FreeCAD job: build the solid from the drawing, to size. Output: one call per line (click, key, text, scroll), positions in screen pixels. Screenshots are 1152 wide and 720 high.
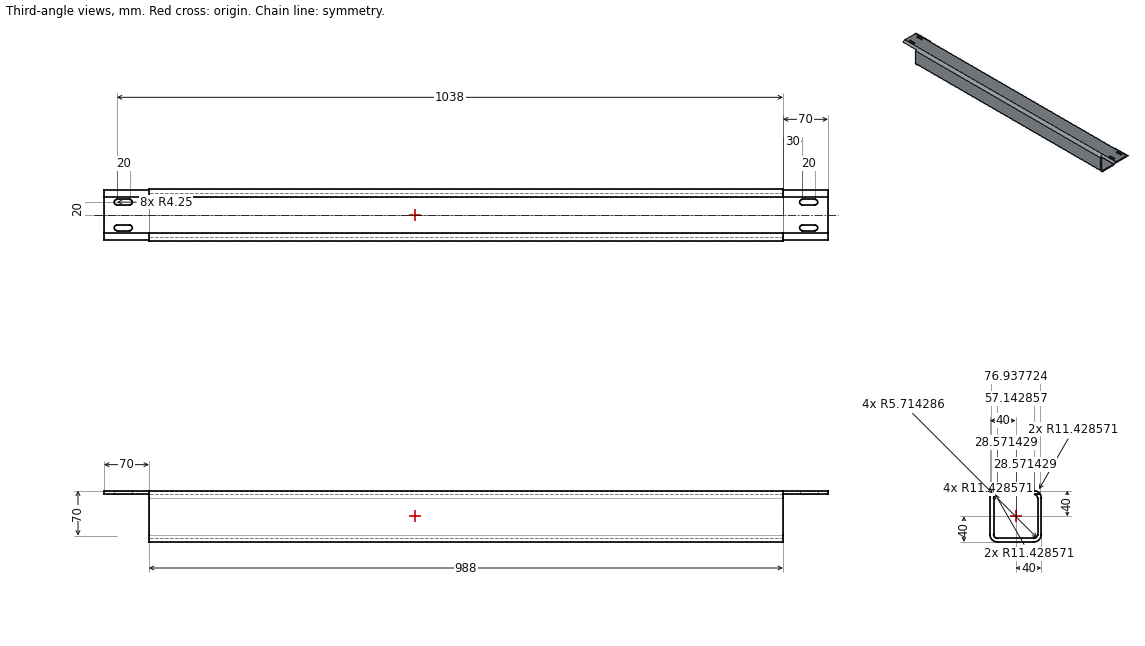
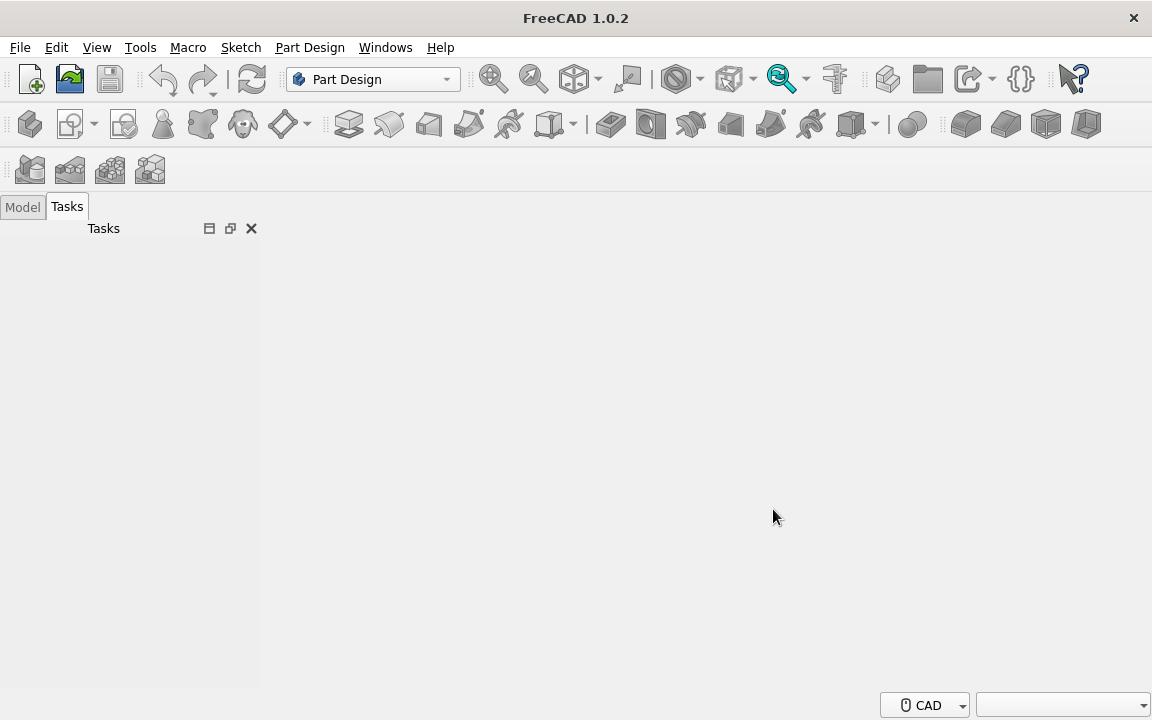
key(ctrl+n)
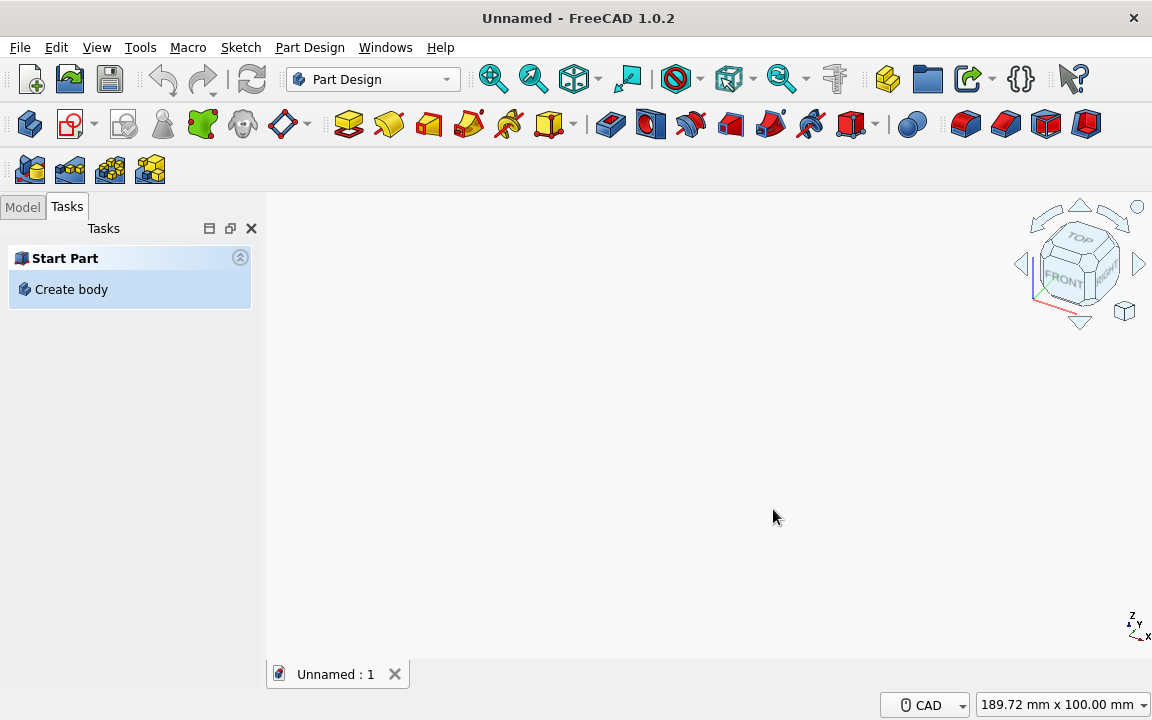
click(30, 124)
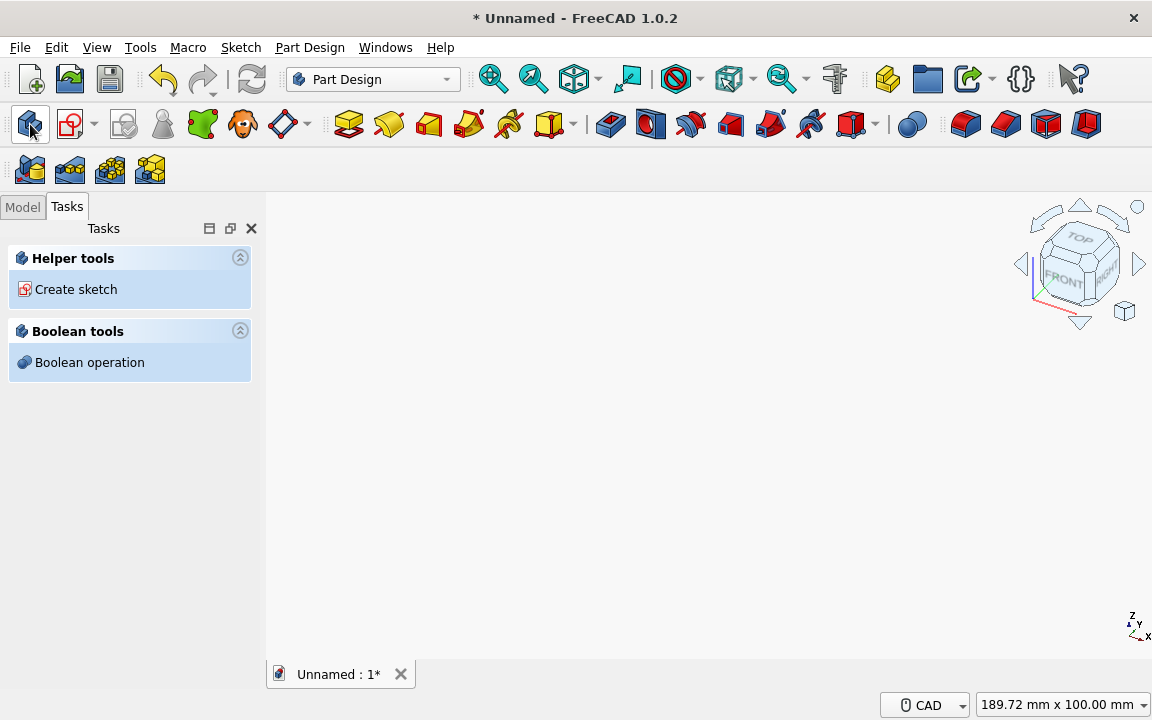
click(23, 206)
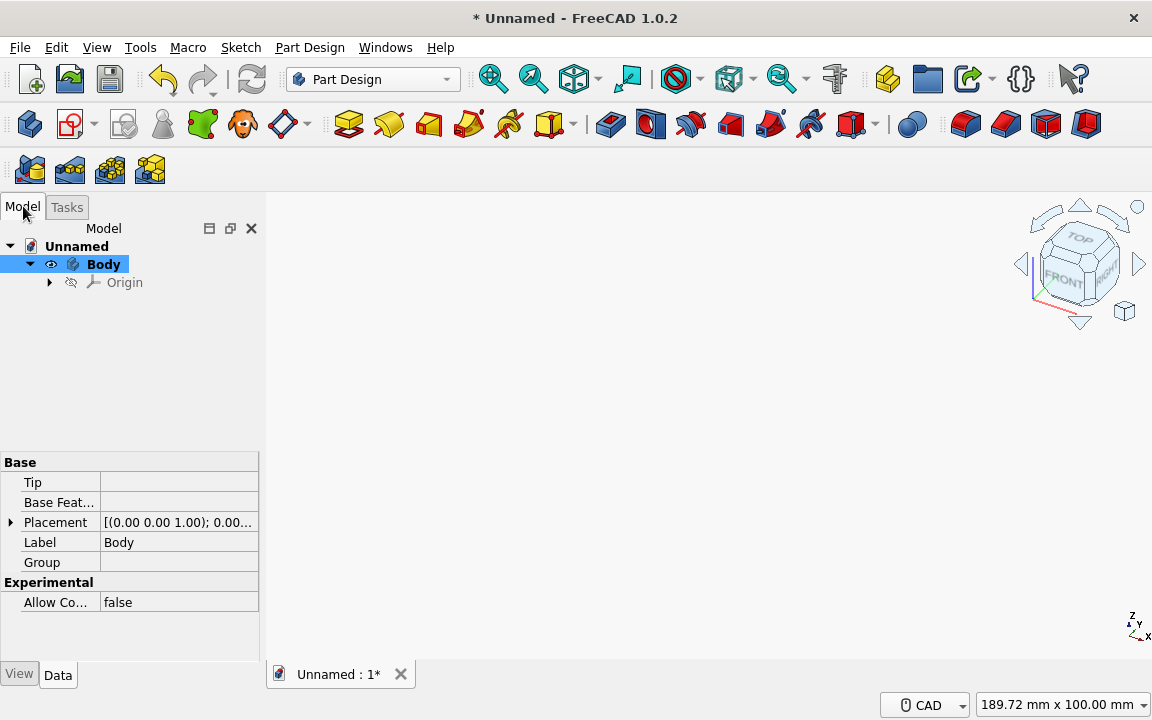
click(50, 282)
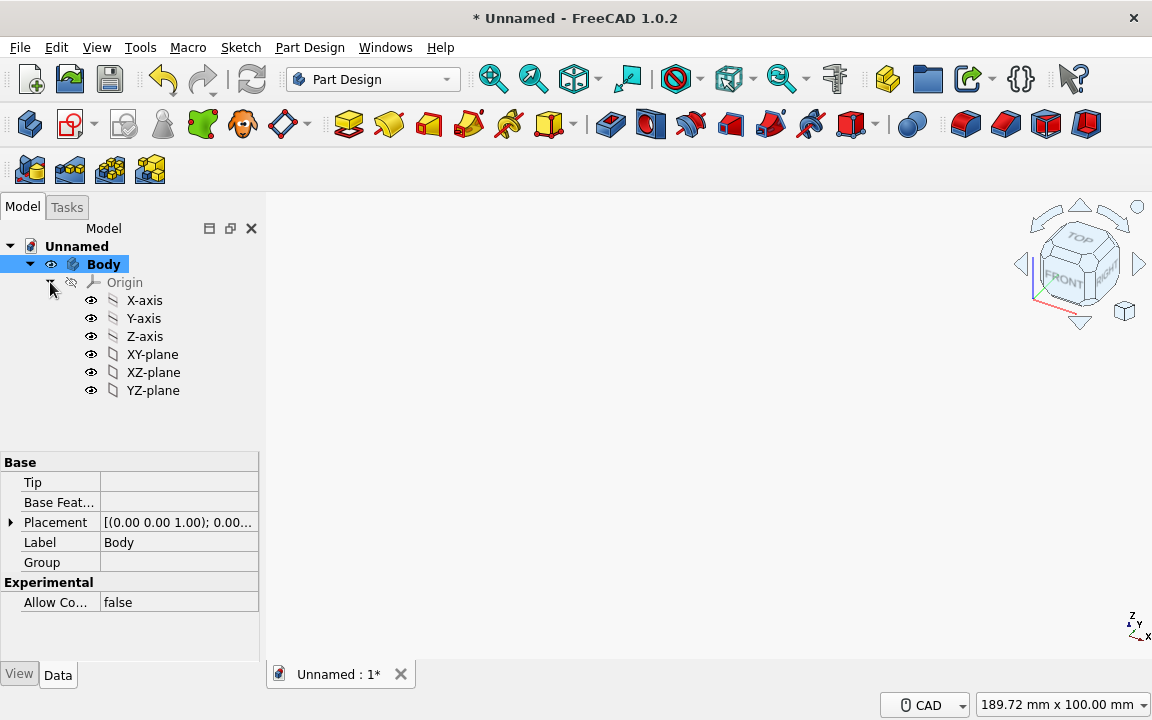
click(136, 390)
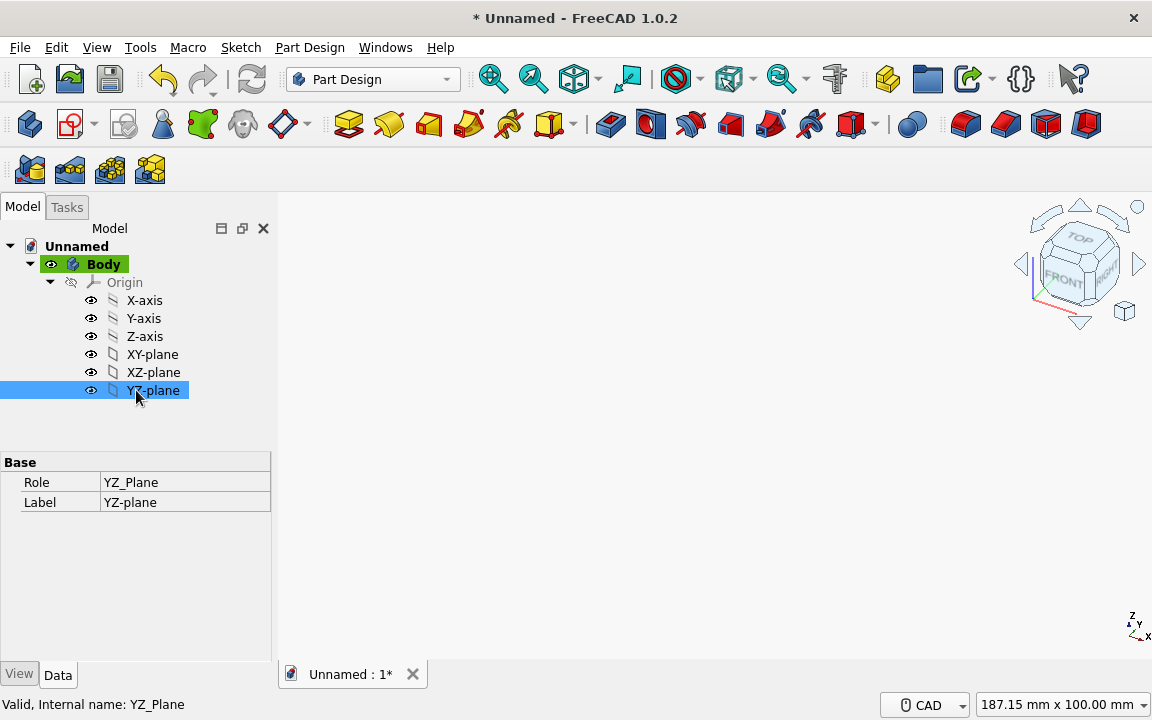
click(284, 124)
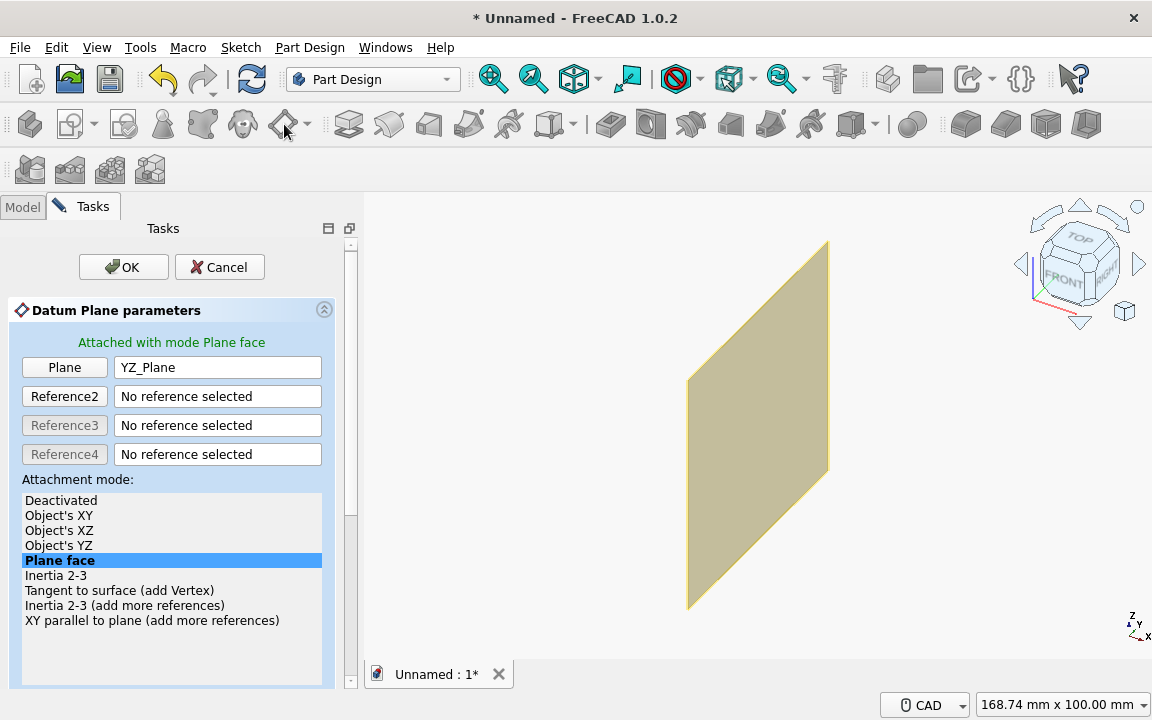
scroll(351, 463, down, 3)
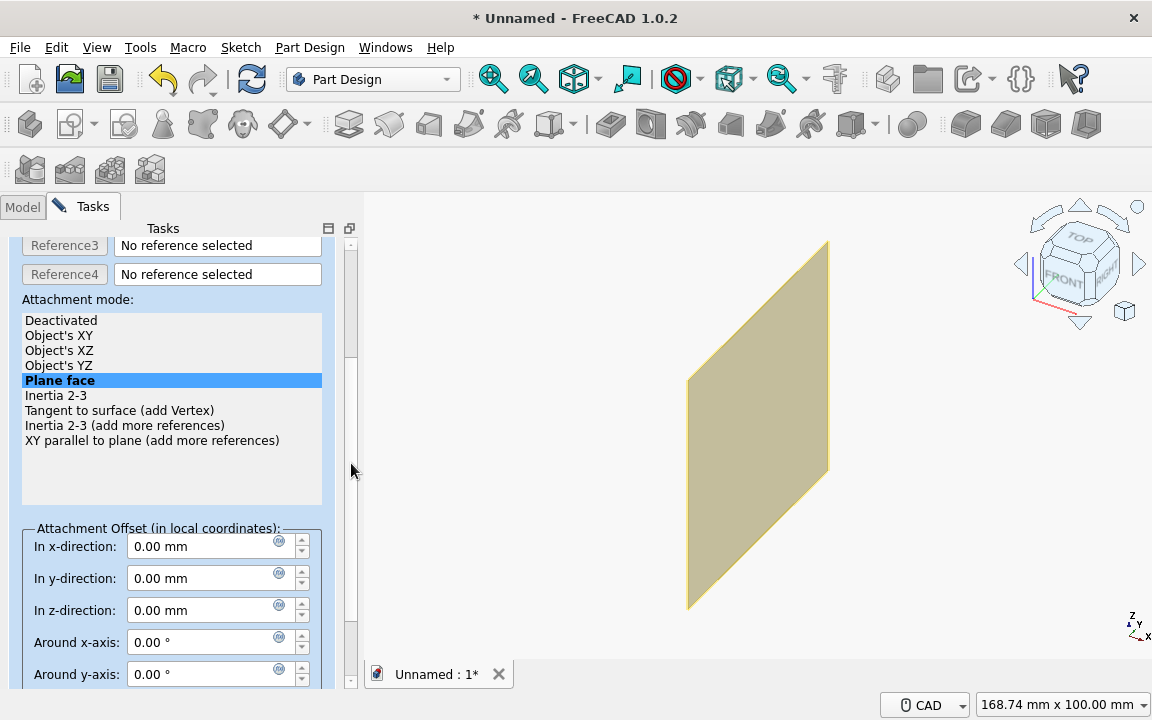
triple_click(210, 610)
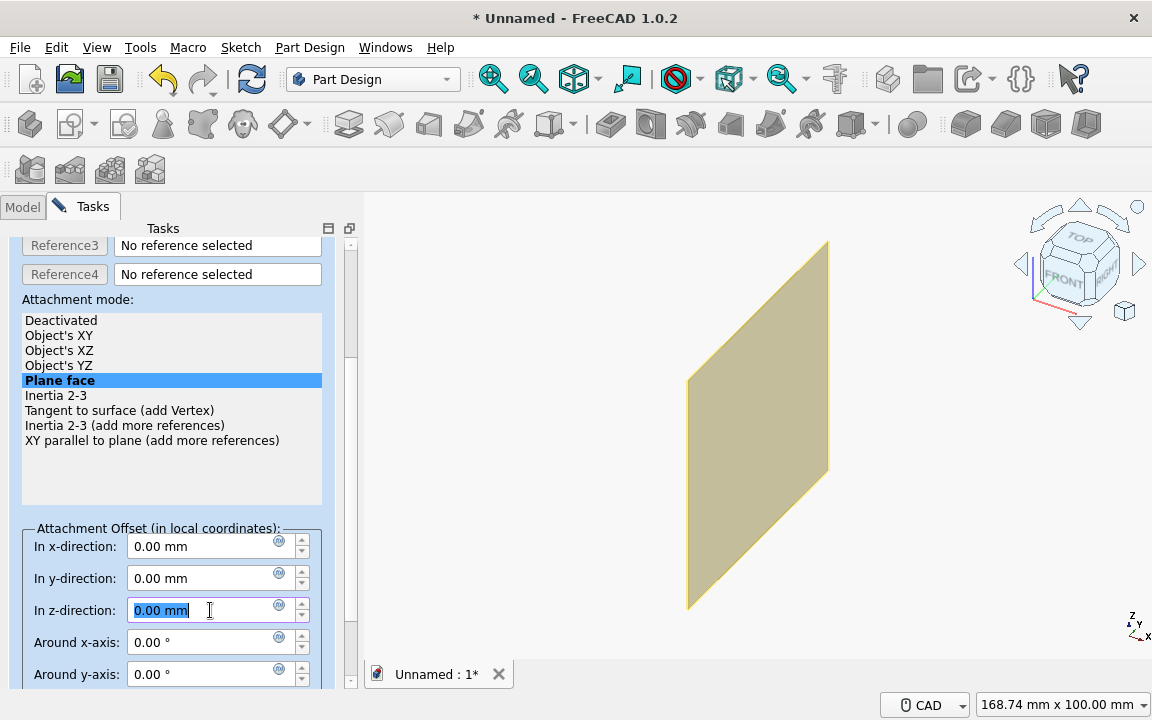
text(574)
key(Tab)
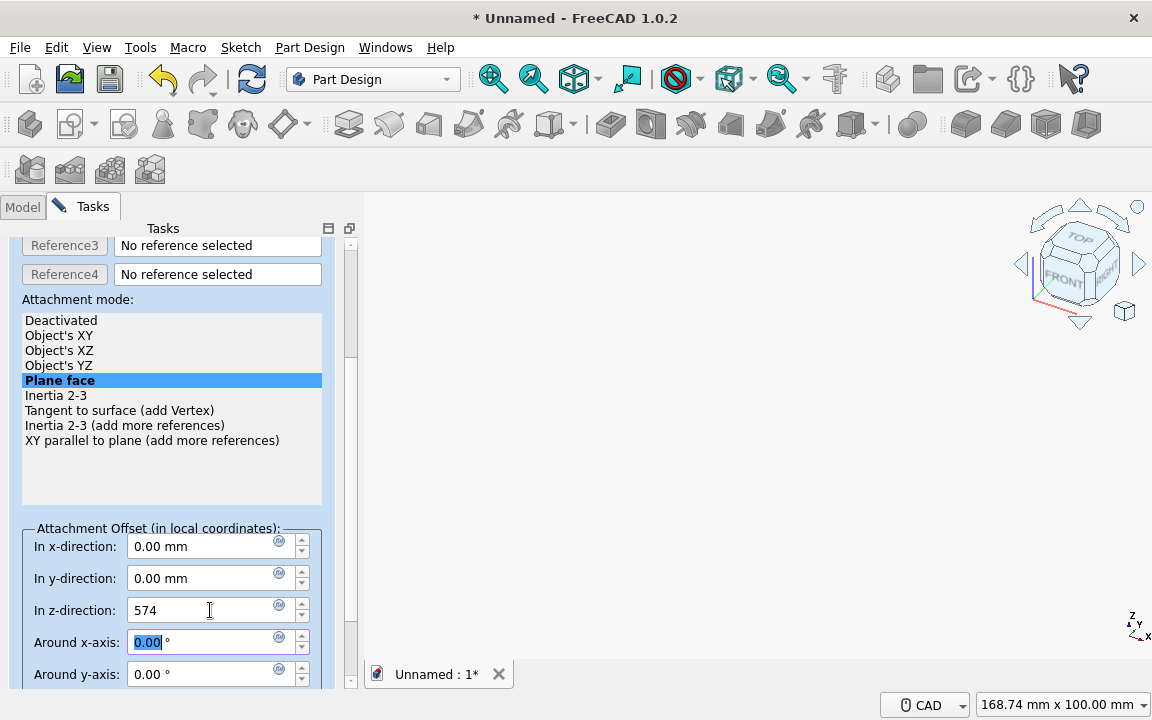
scroll(351, 463, up, 4)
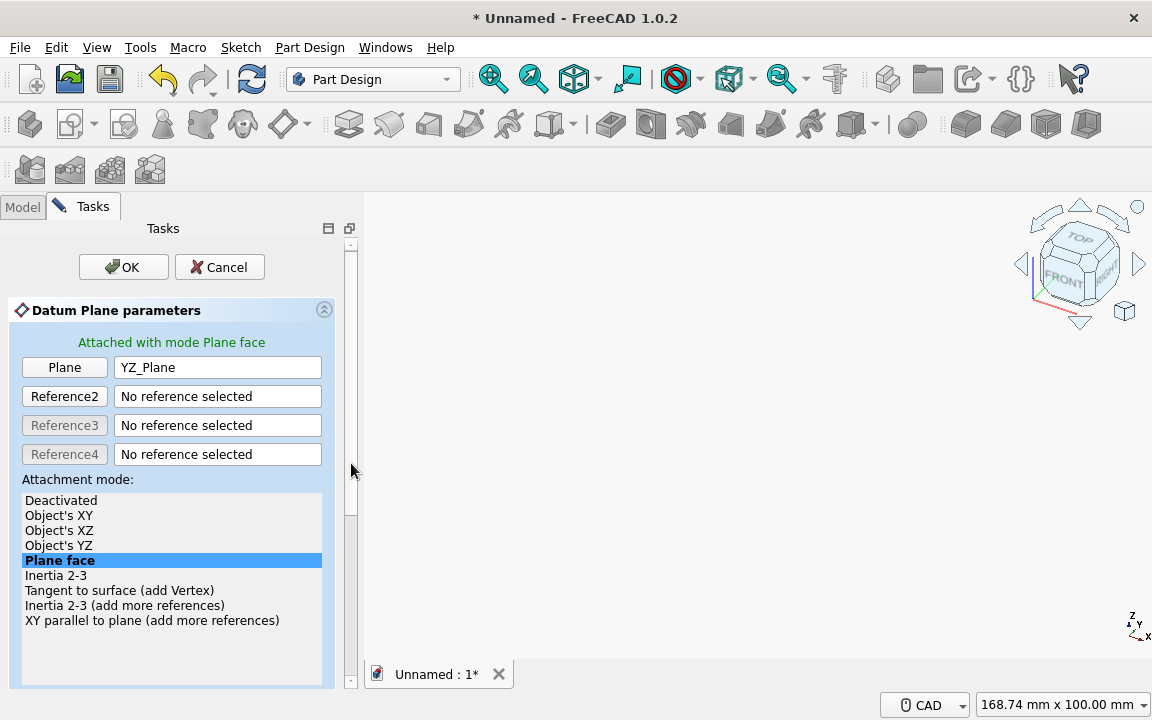
click(124, 267)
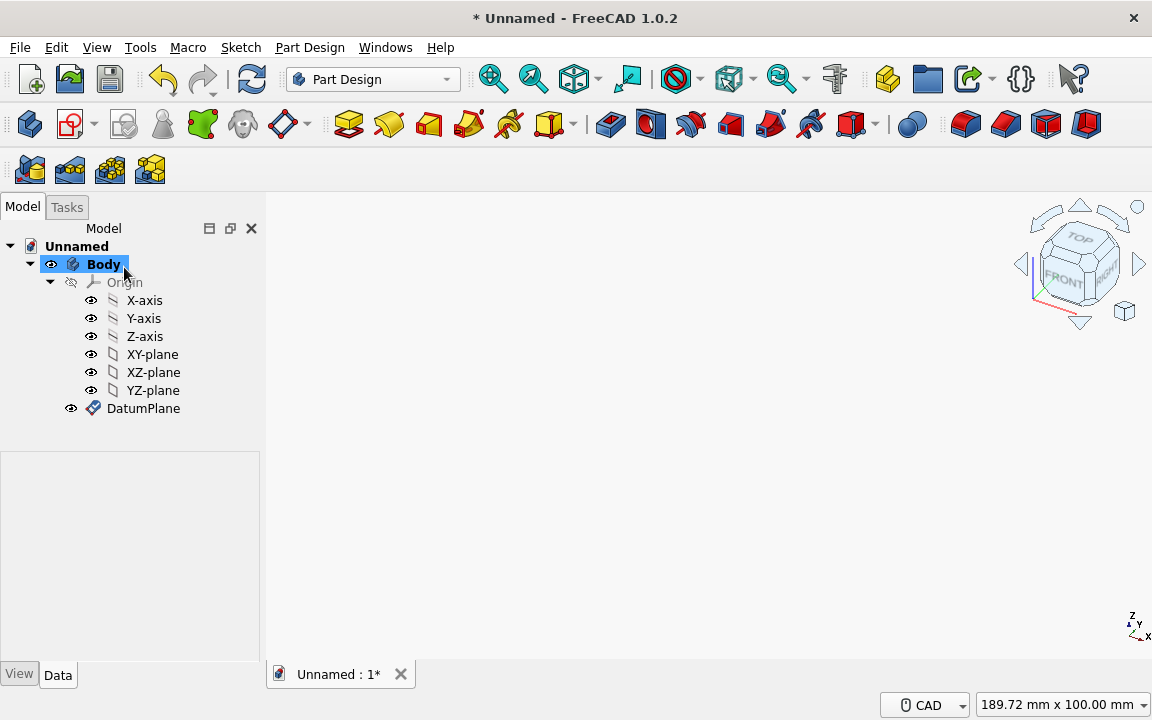
click(116, 408)